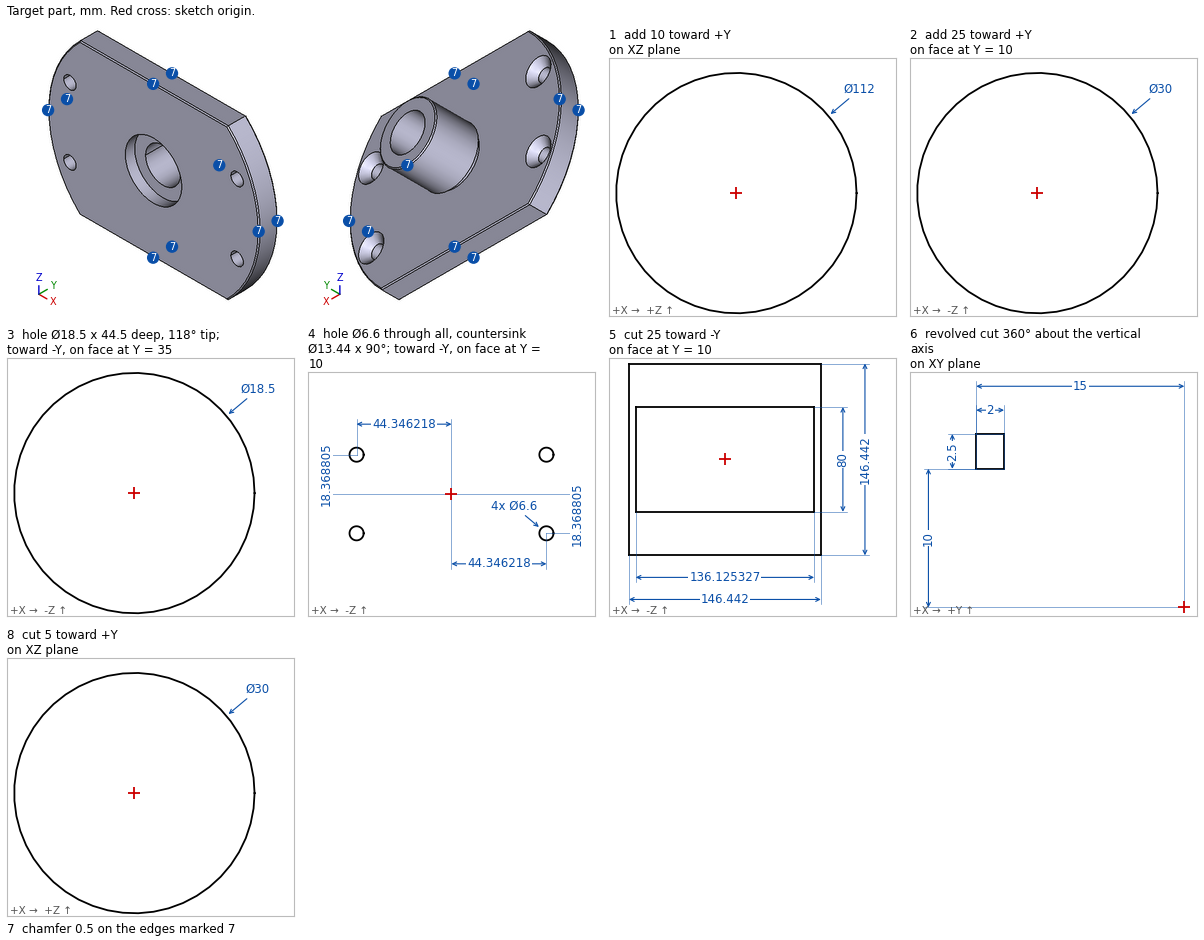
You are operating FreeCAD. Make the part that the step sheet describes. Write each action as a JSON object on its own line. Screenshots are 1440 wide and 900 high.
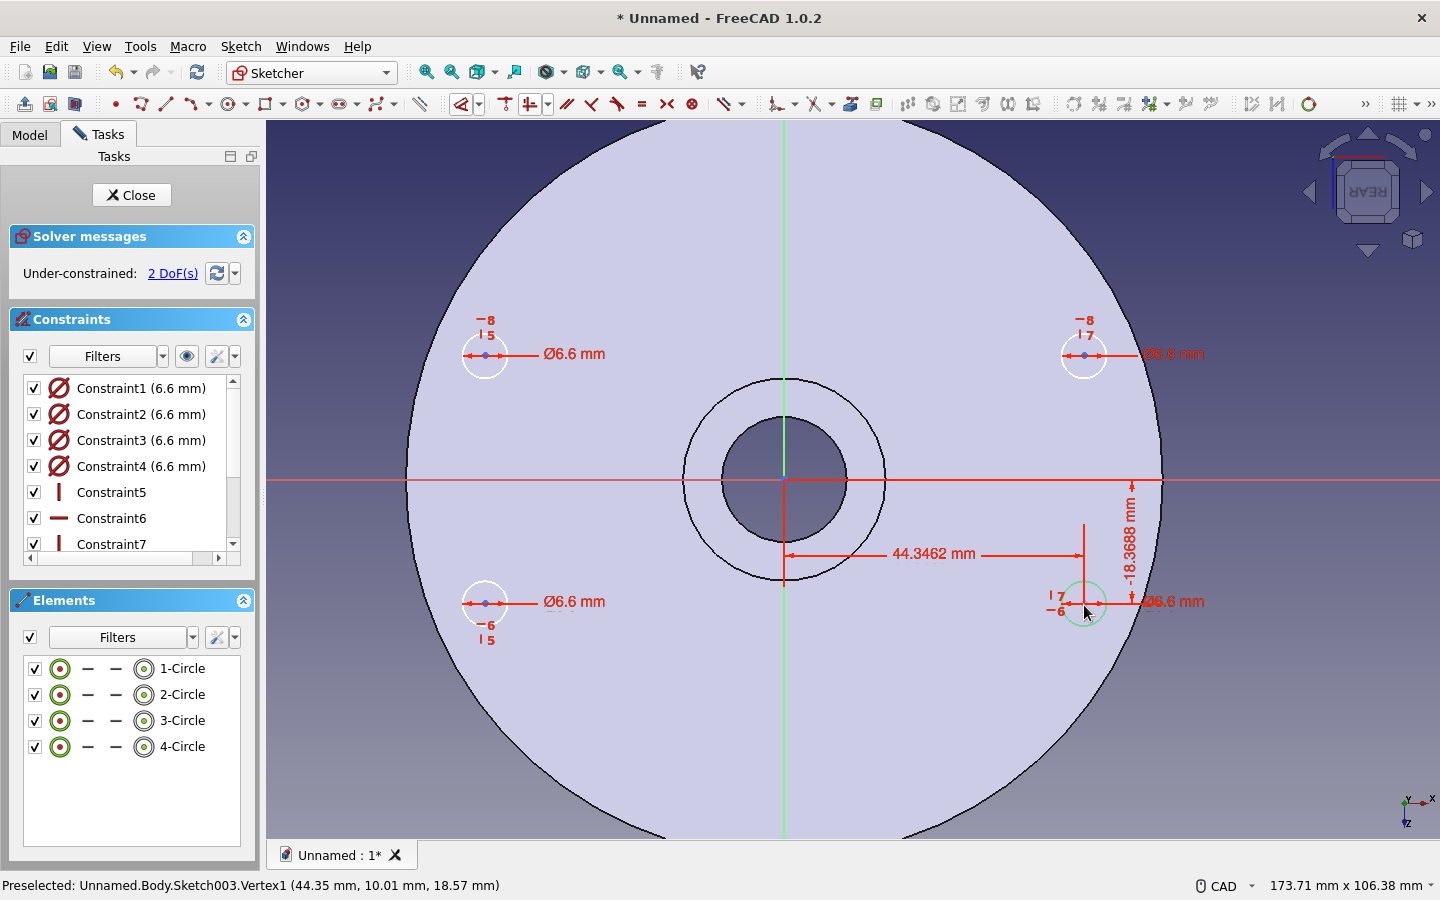
{"action": "left_click", "coordinate": [485, 356]}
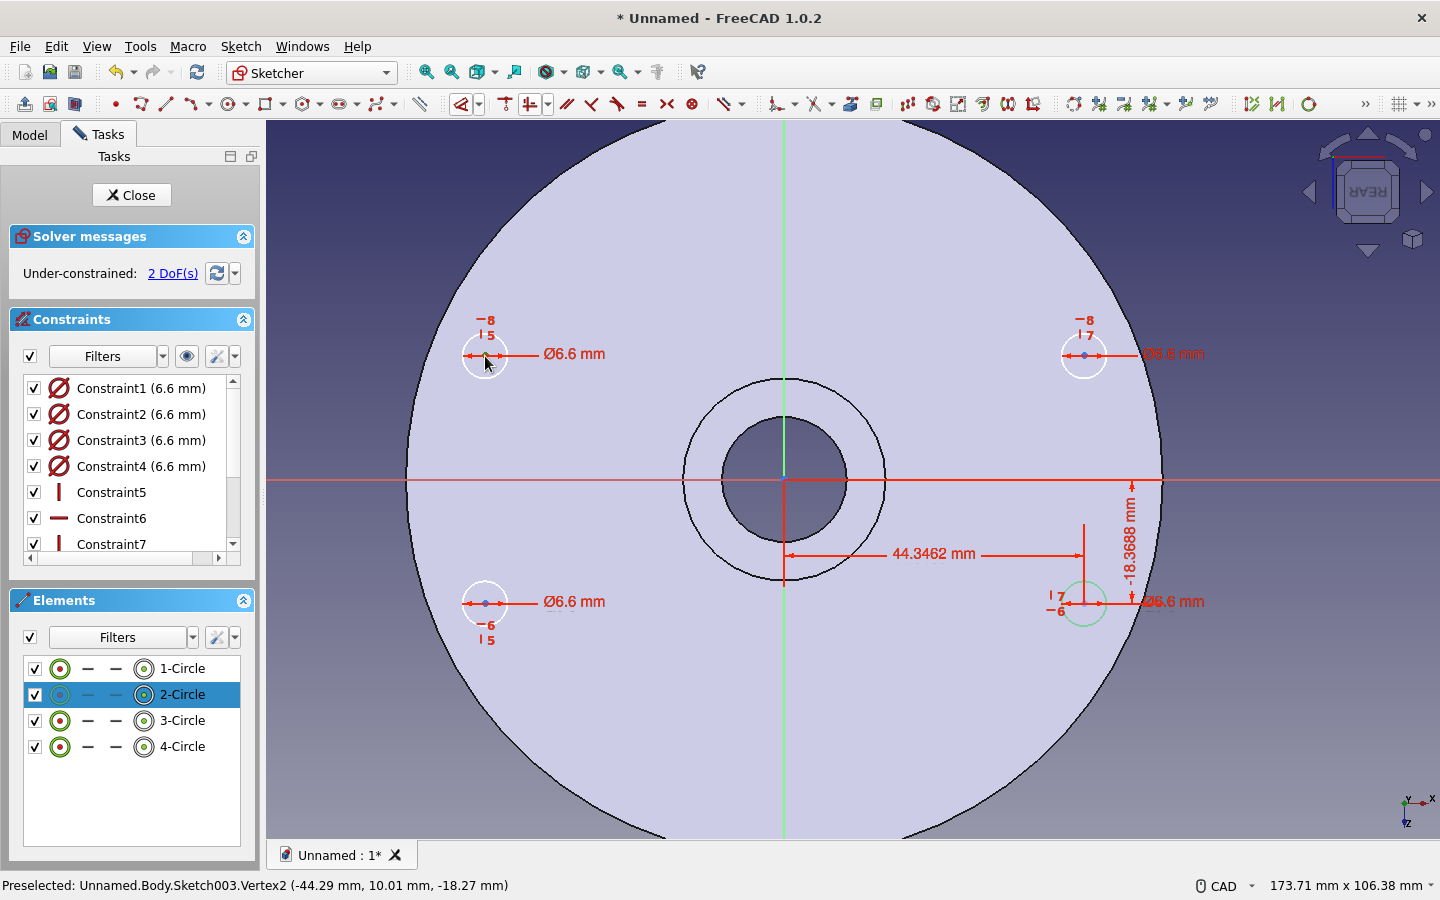
{"action": "left_click", "coordinate": [478, 104]}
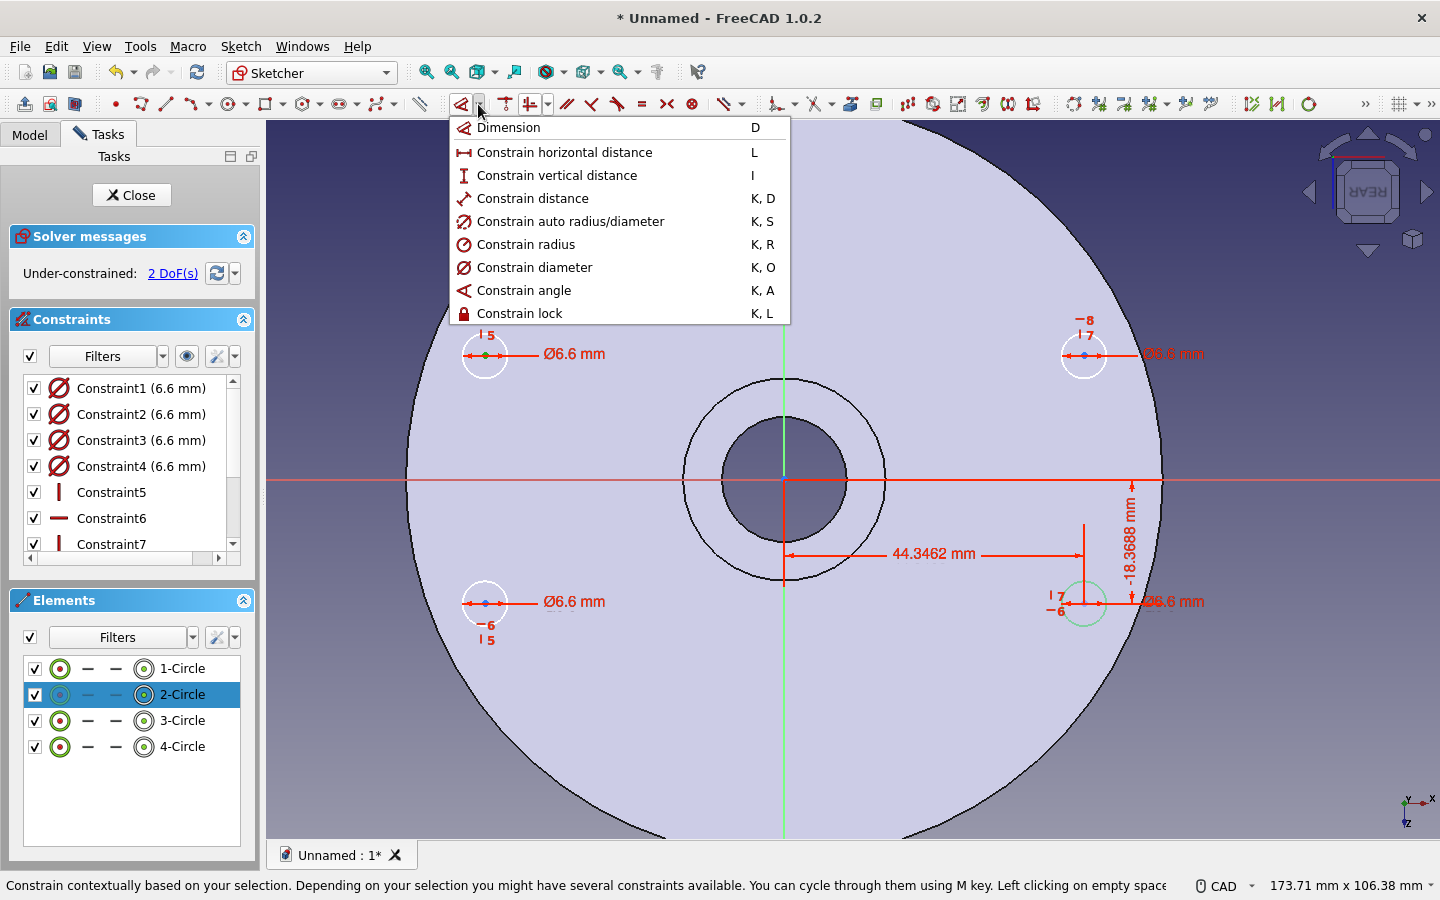
{"action": "left_click", "coordinate": [620, 152]}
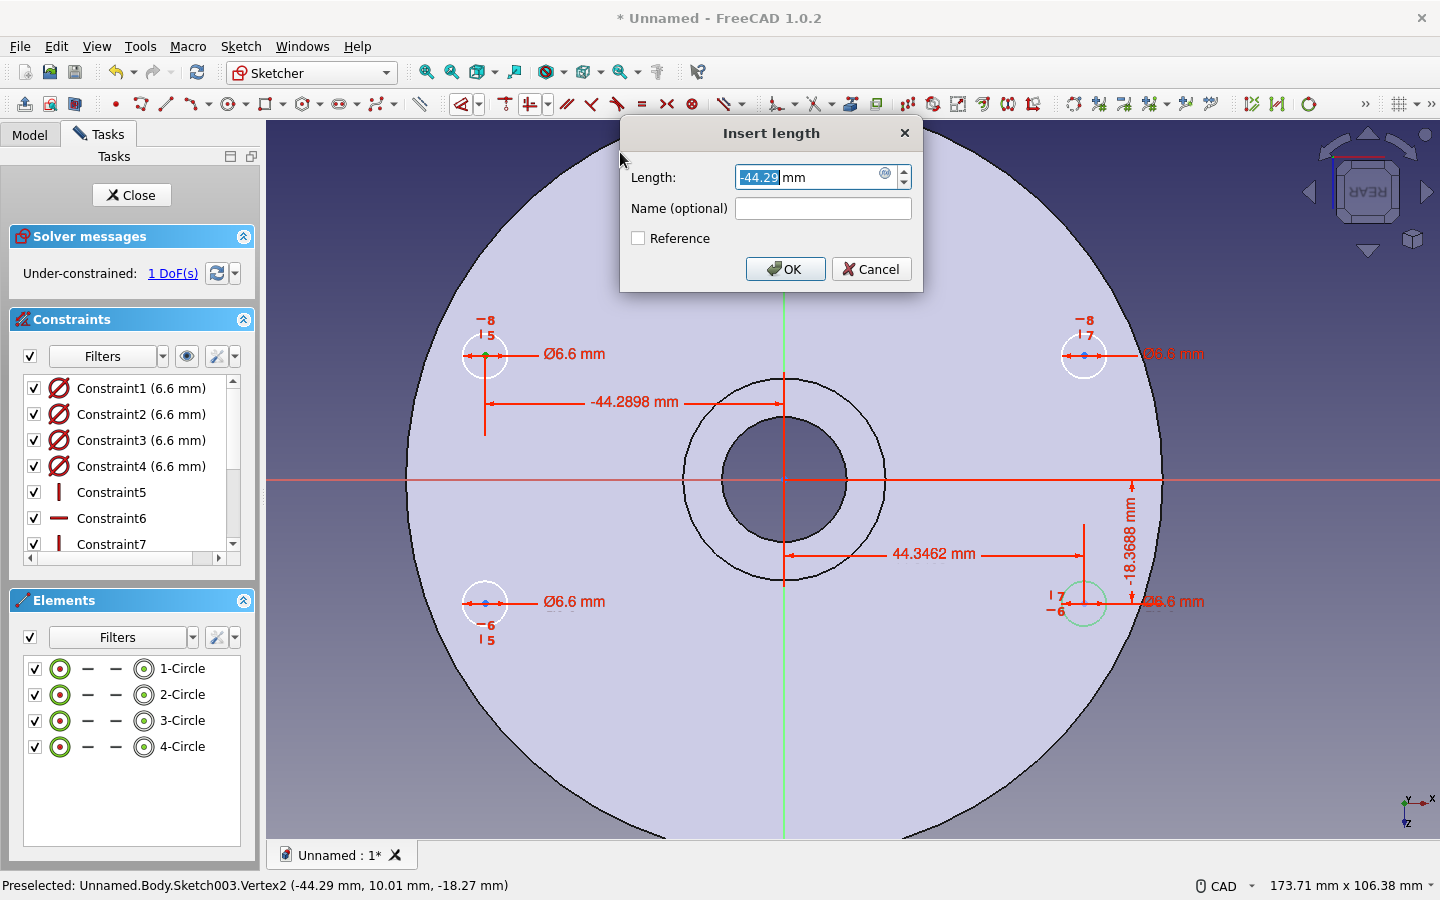
{"action": "type", "text": "-44.346218"}
{"action": "key", "text": "Return"}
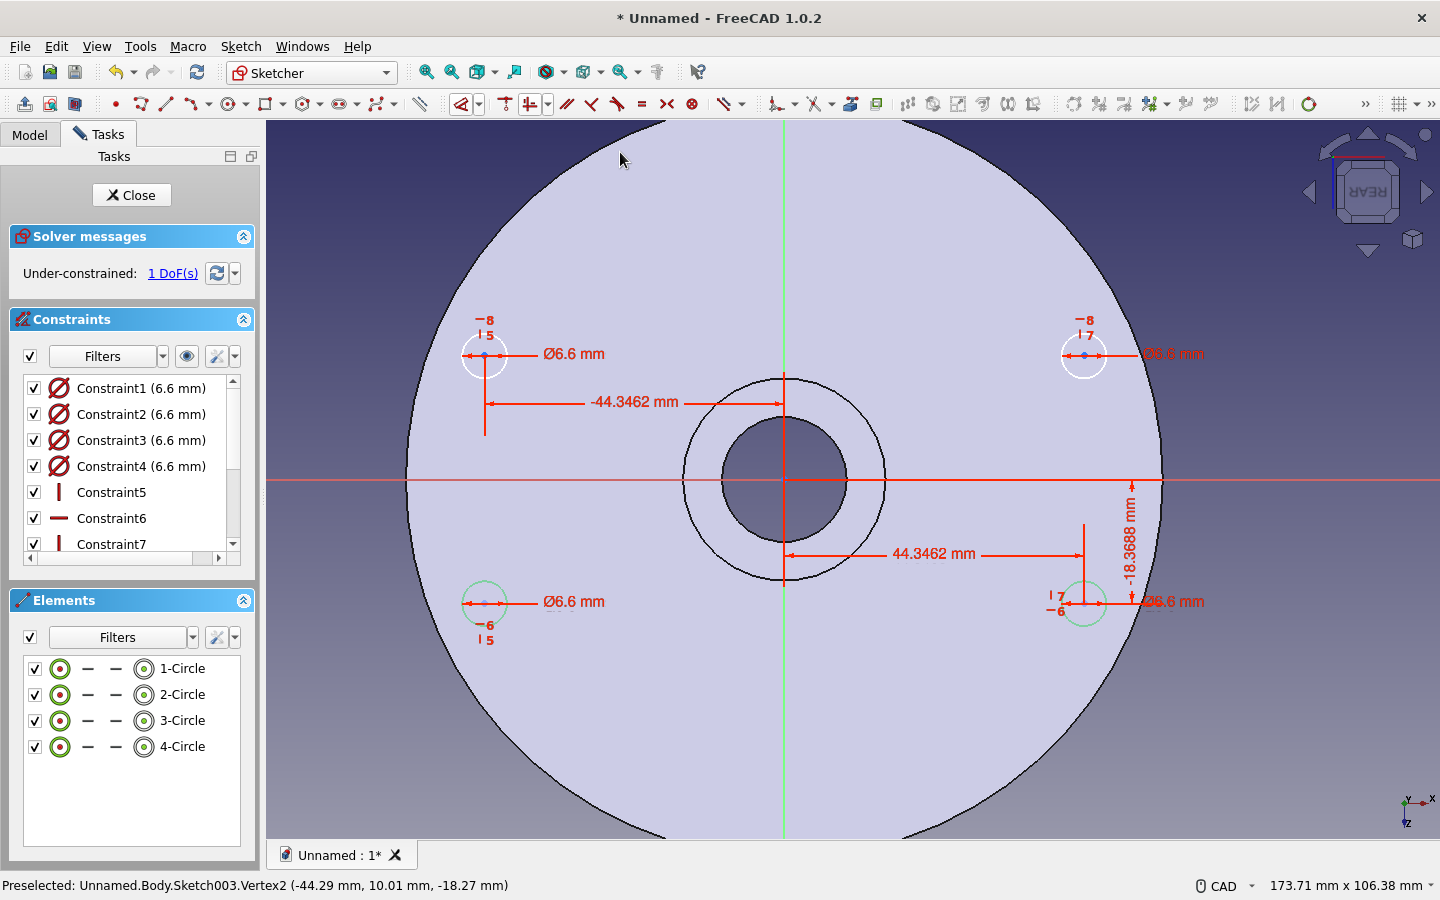
{"action": "left_click", "coordinate": [485, 356]}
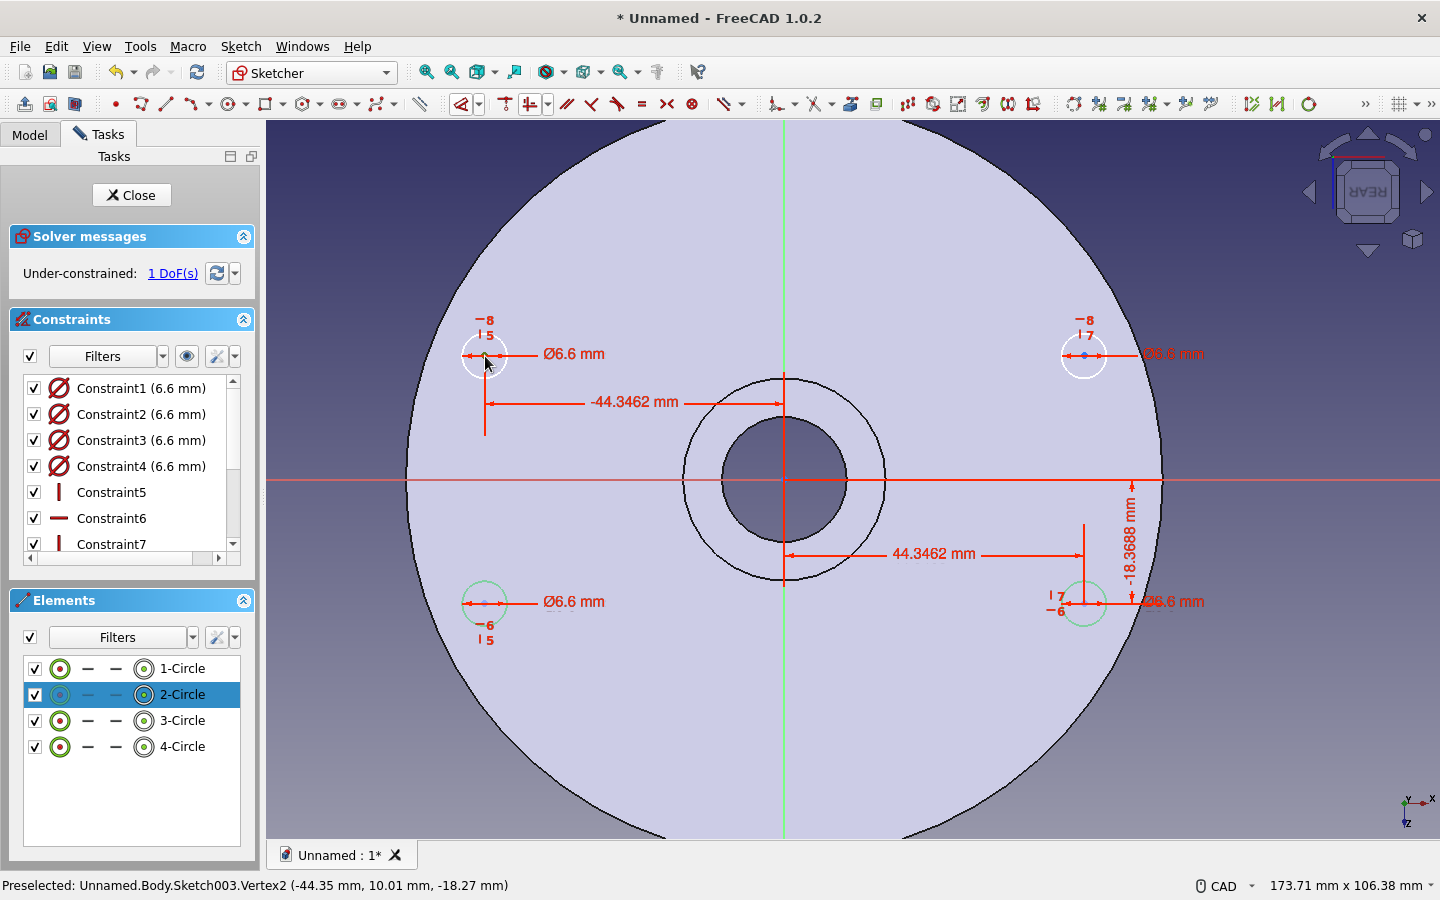
{"action": "key", "text": "i"}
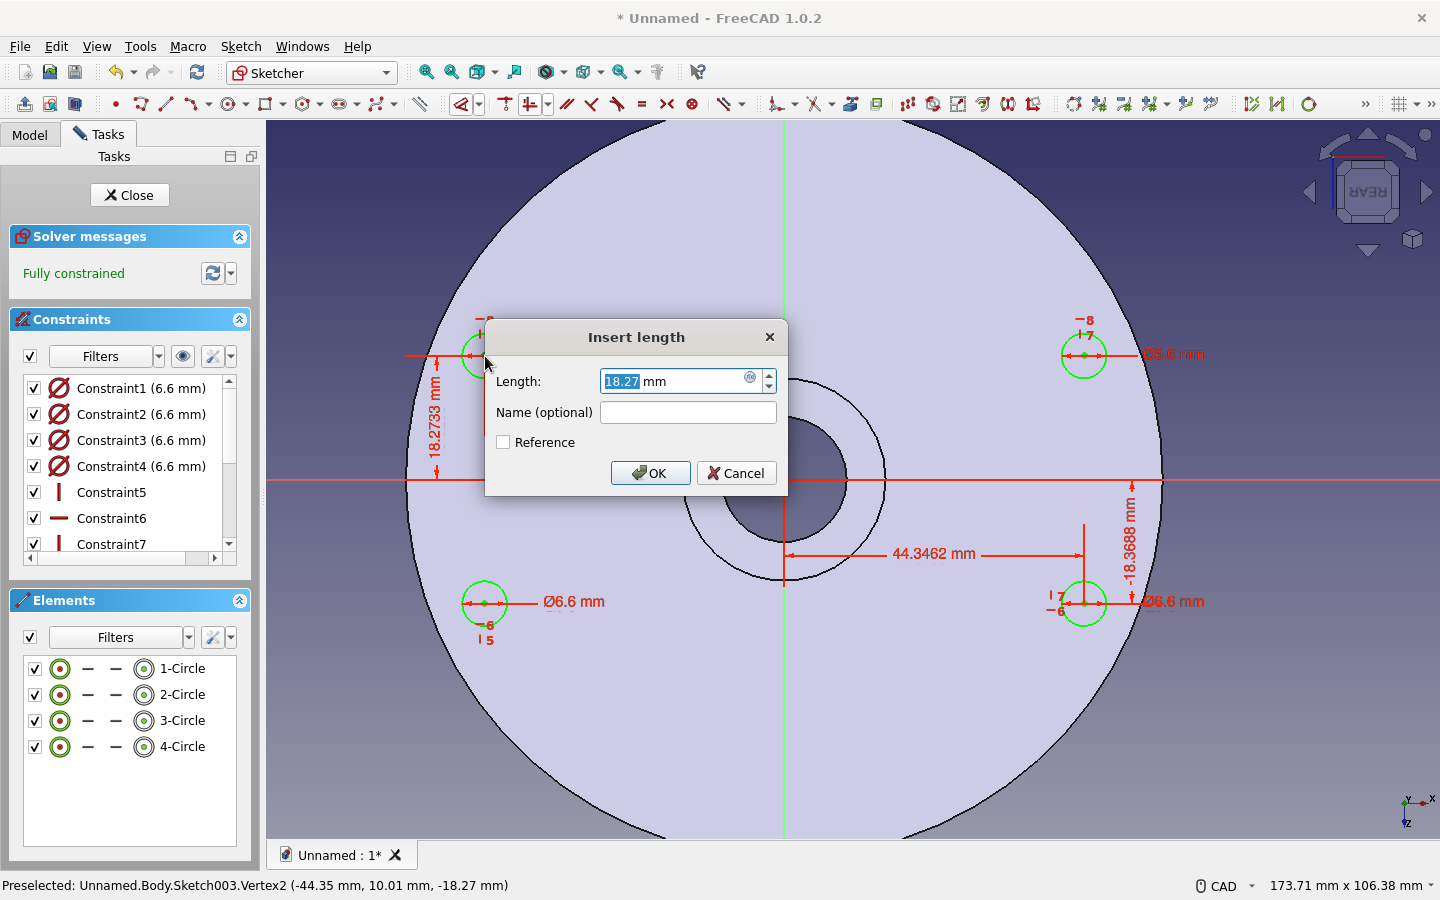
{"action": "type", "text": "18.368805"}
{"action": "key", "text": "Return"}